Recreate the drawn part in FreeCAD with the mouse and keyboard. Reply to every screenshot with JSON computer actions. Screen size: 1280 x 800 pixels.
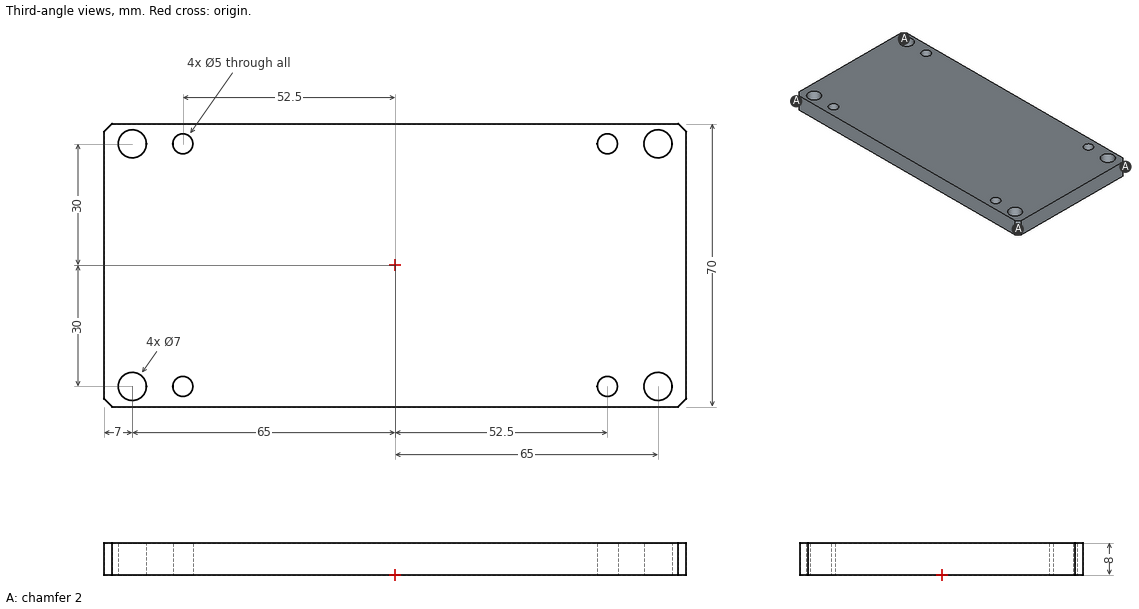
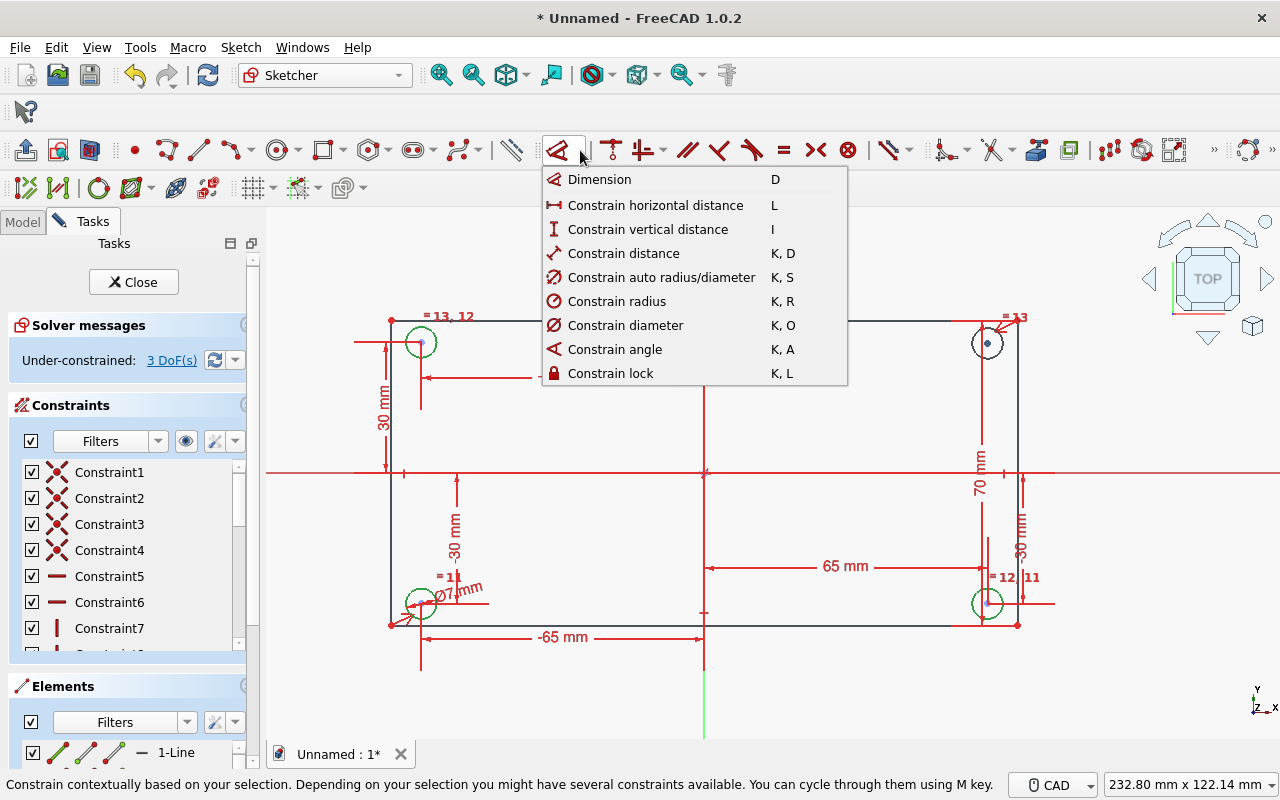
{"action": "left_click", "coordinate": [695, 205]}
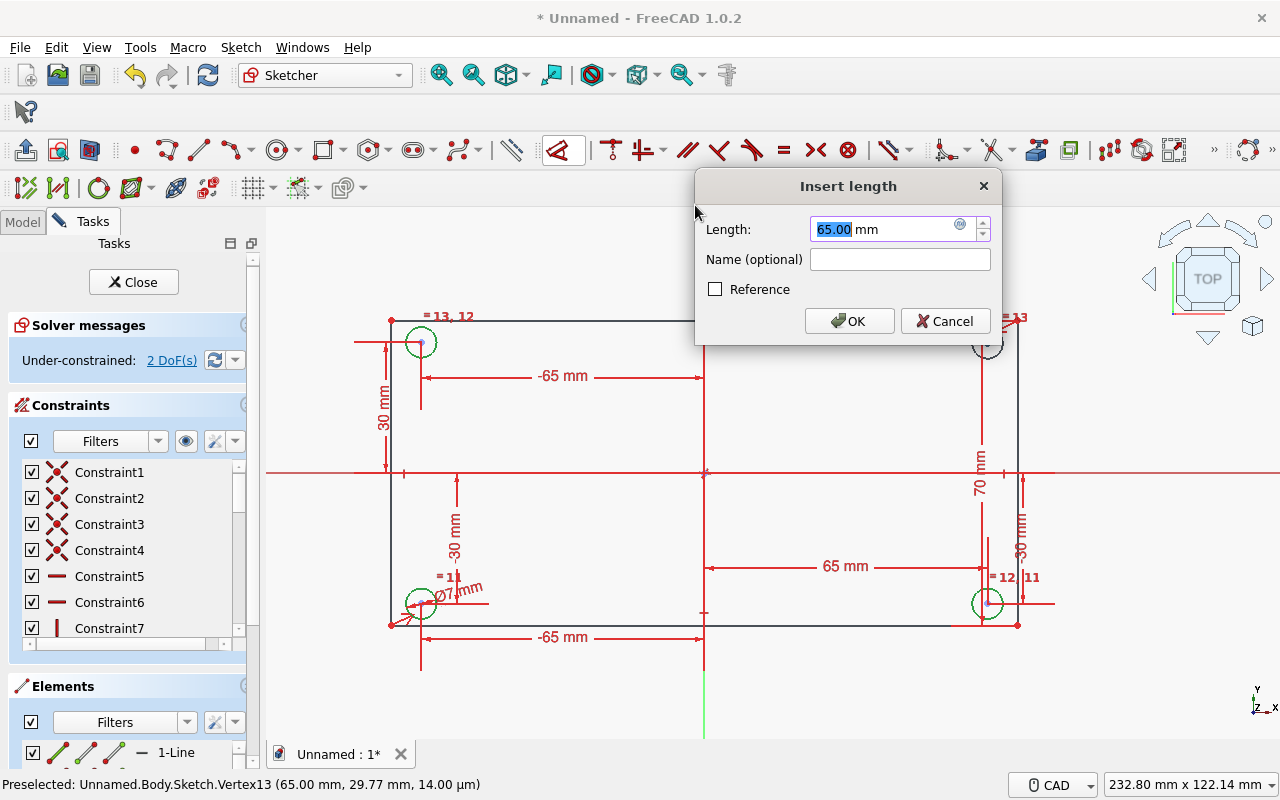
{"action": "type", "text": "65"}
{"action": "key", "text": "Return"}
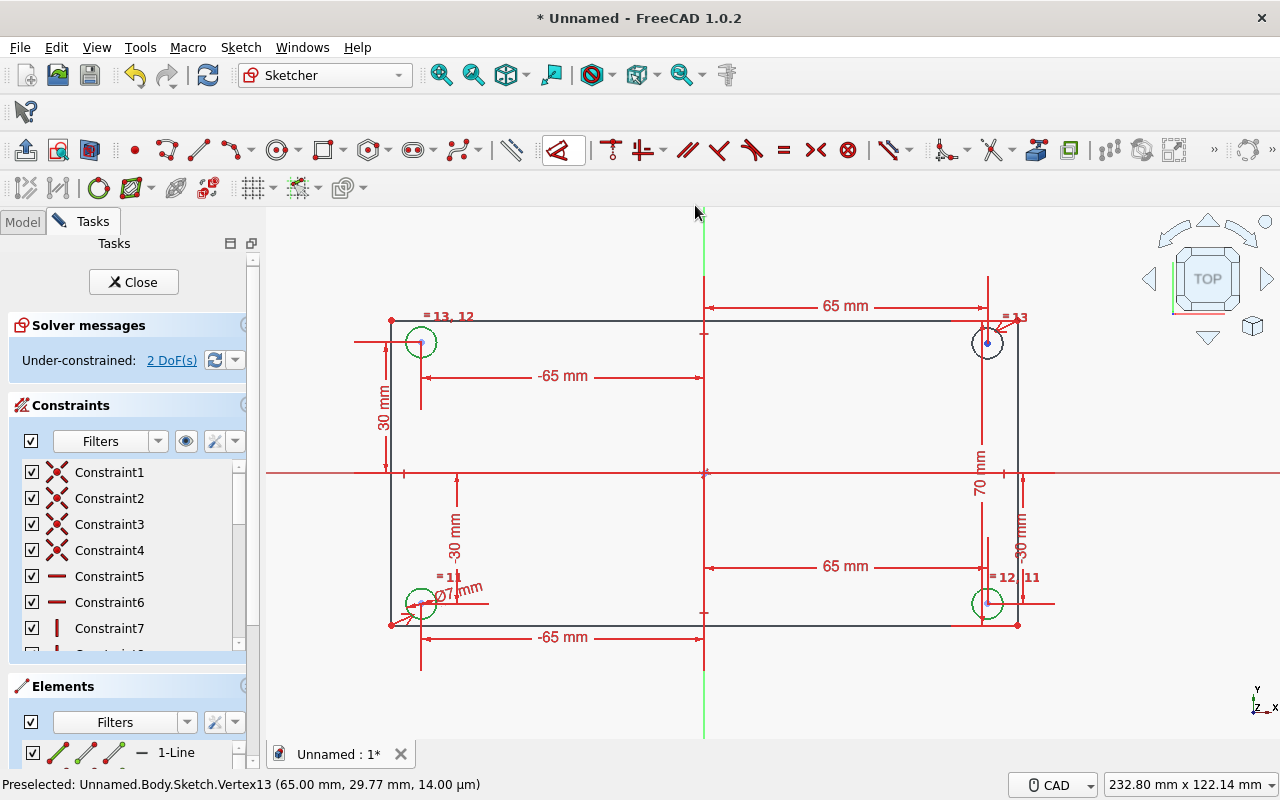
{"action": "left_click", "coordinate": [988, 343]}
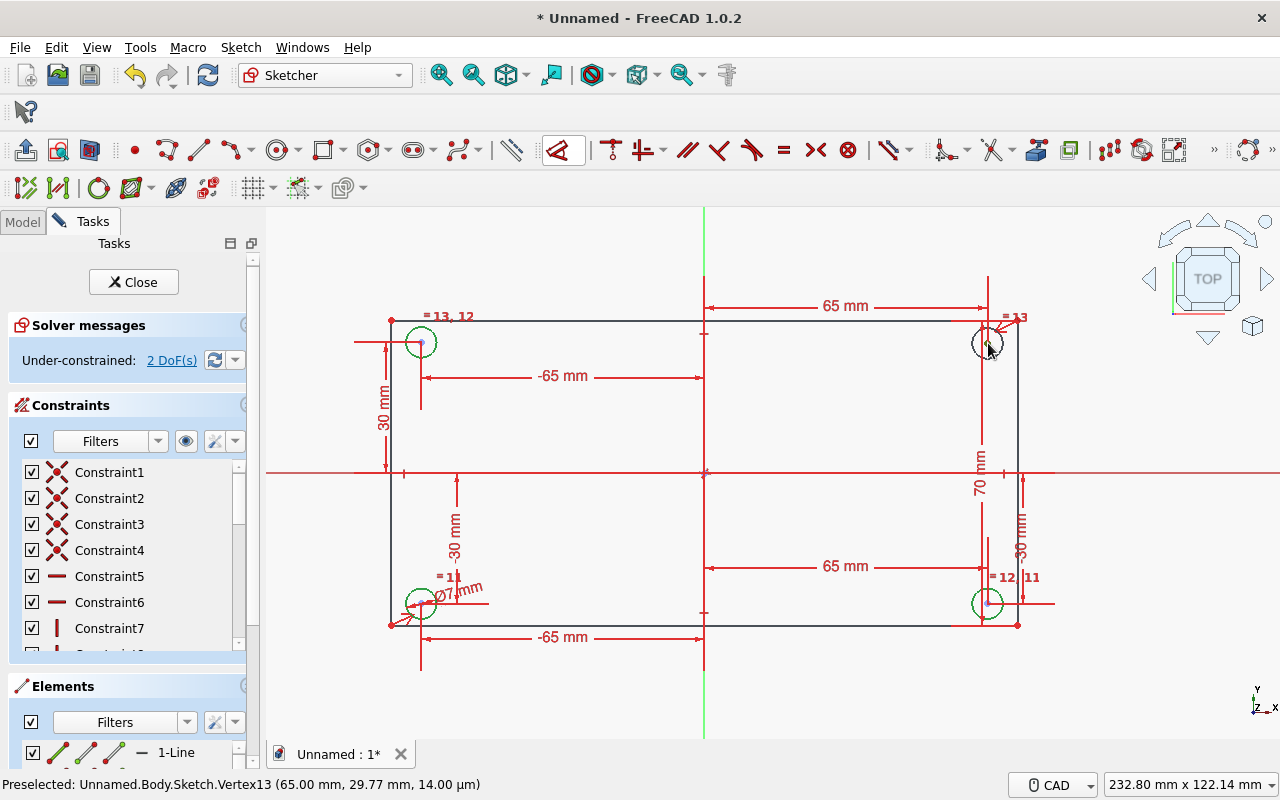
{"action": "key", "text": "i"}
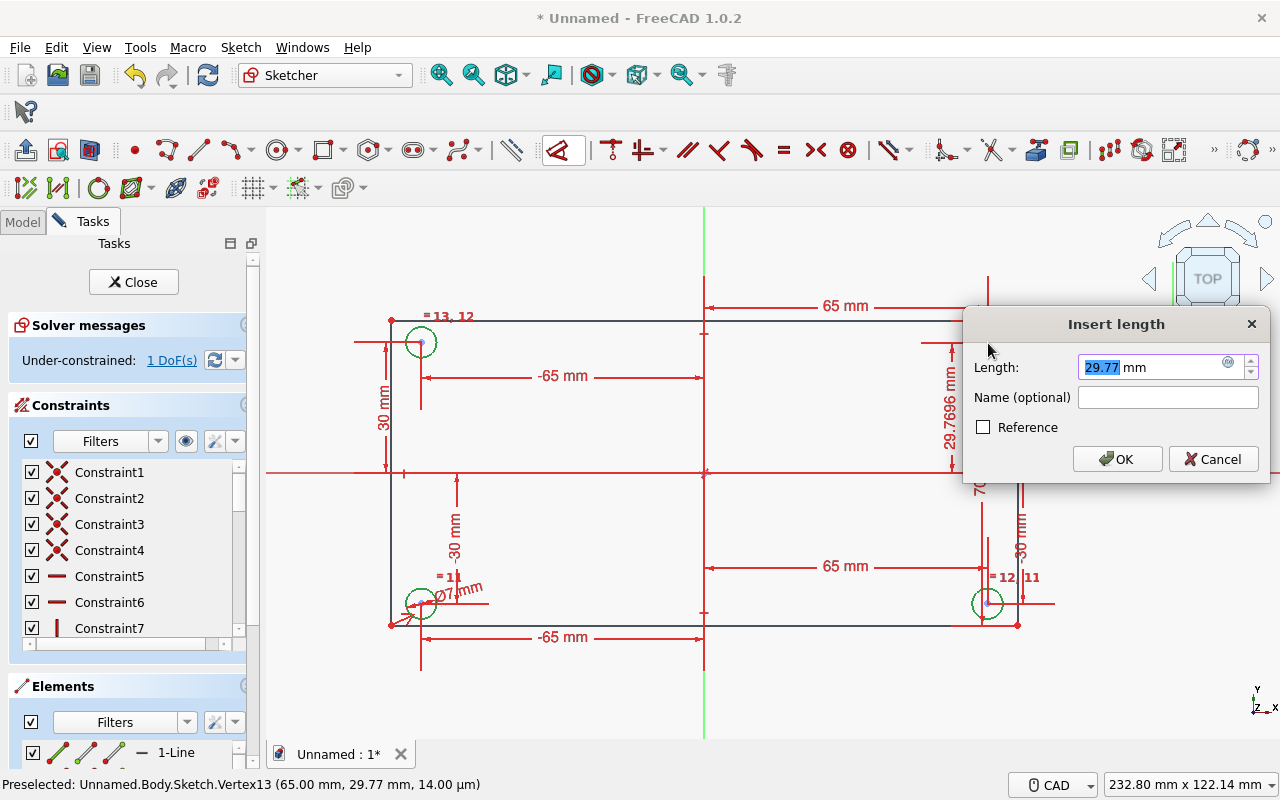
{"action": "type", "text": "30"}
{"action": "key", "text": "Return"}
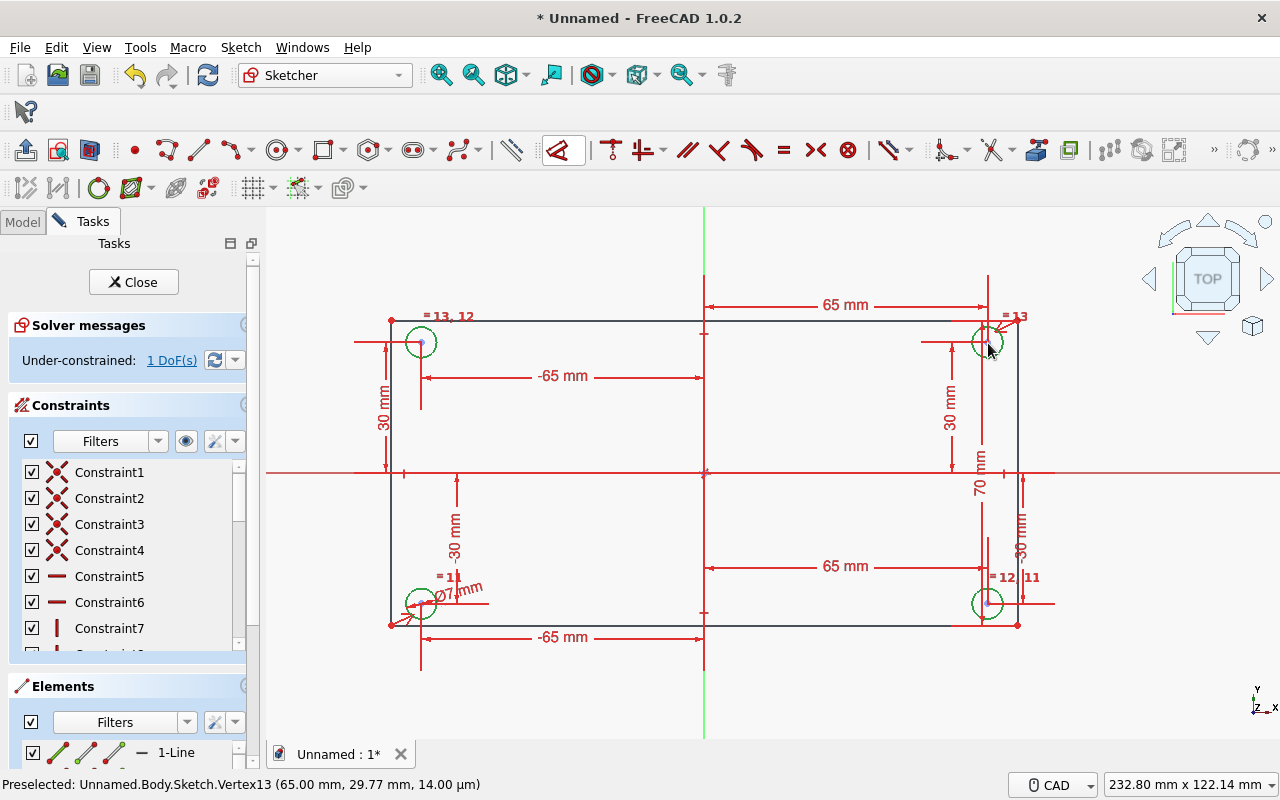
{"action": "scroll", "coordinate": [391, 626], "scroll_direction": "up", "scroll_amount": 2}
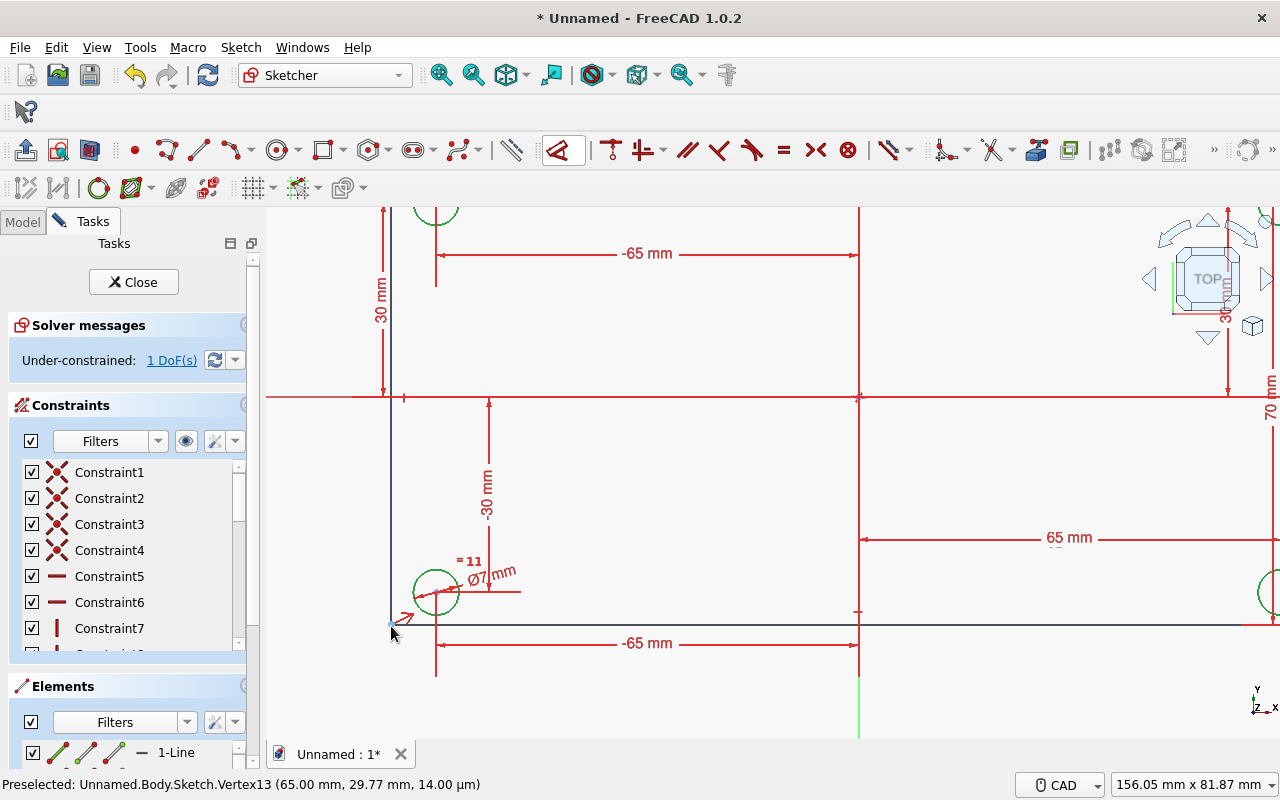
{"action": "left_click", "coordinate": [391, 625]}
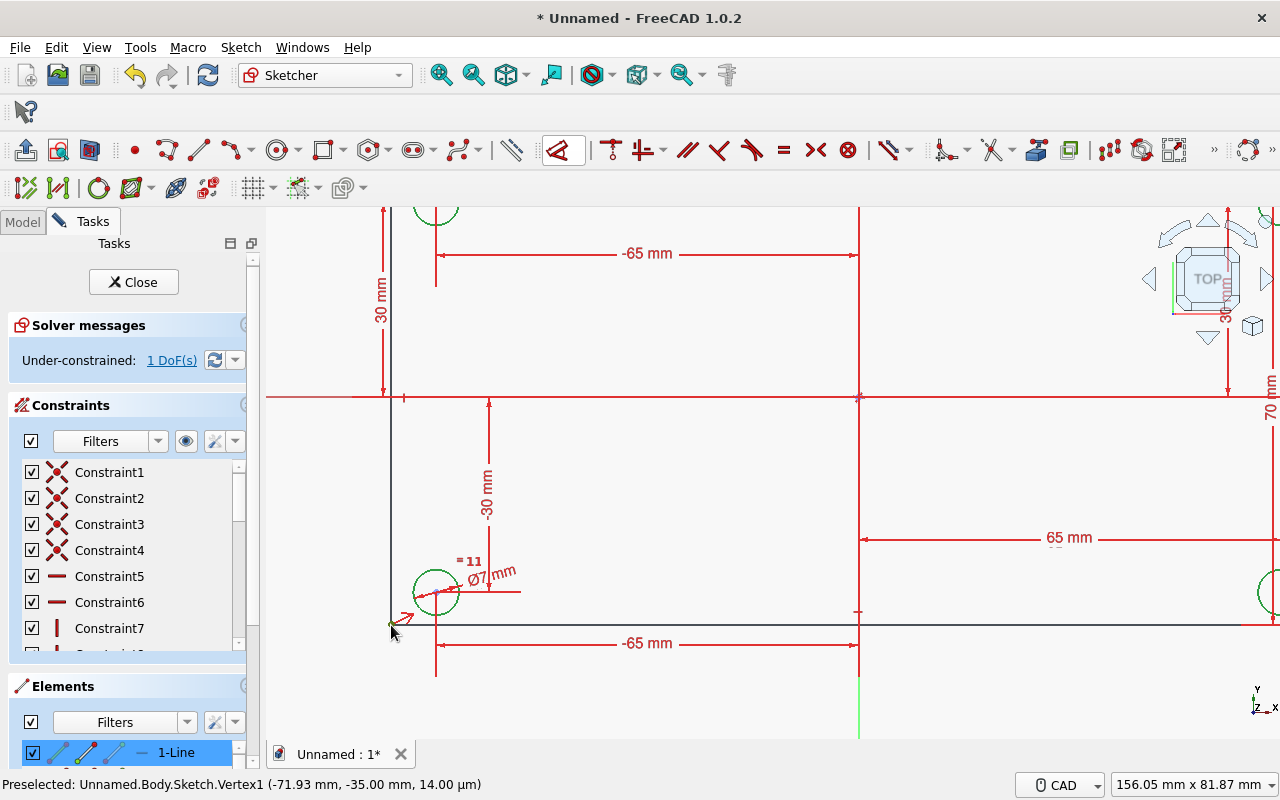
{"action": "left_click", "coordinate": [436, 592]}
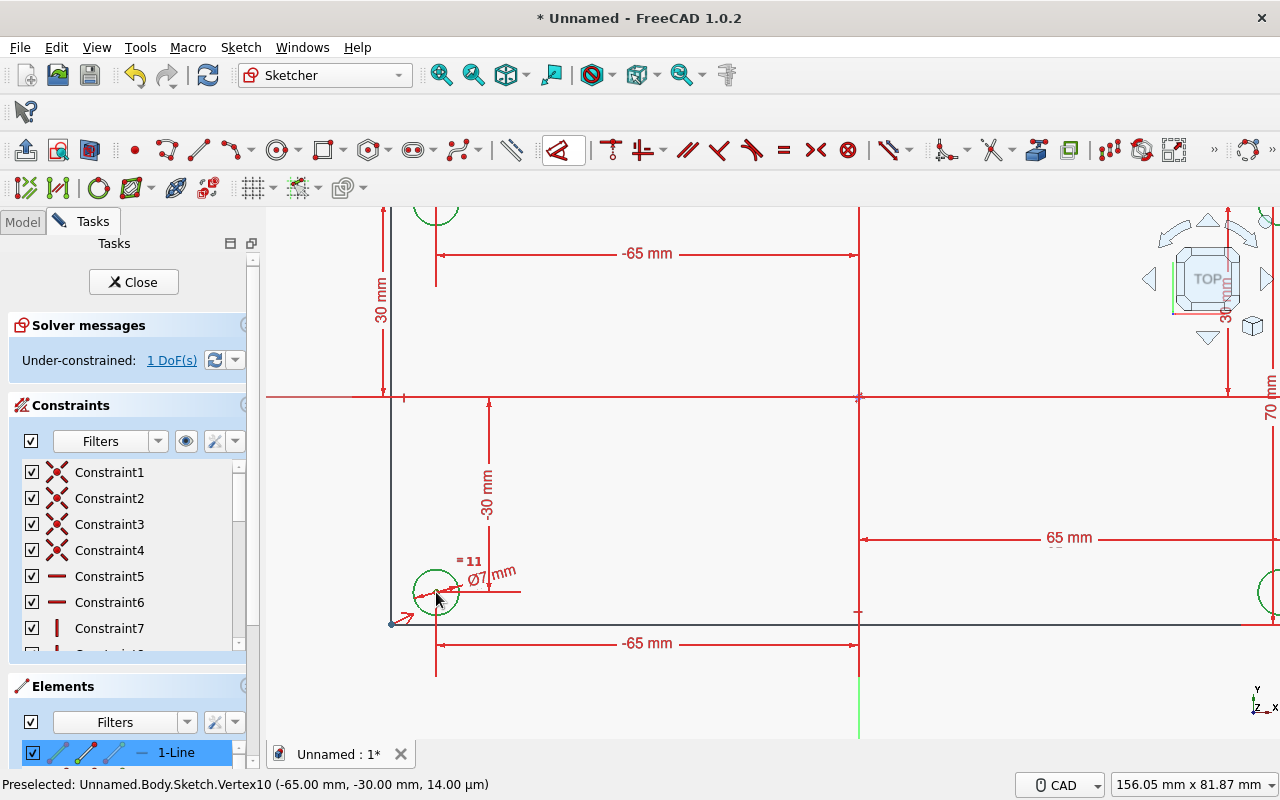
{"action": "key", "text": "l"}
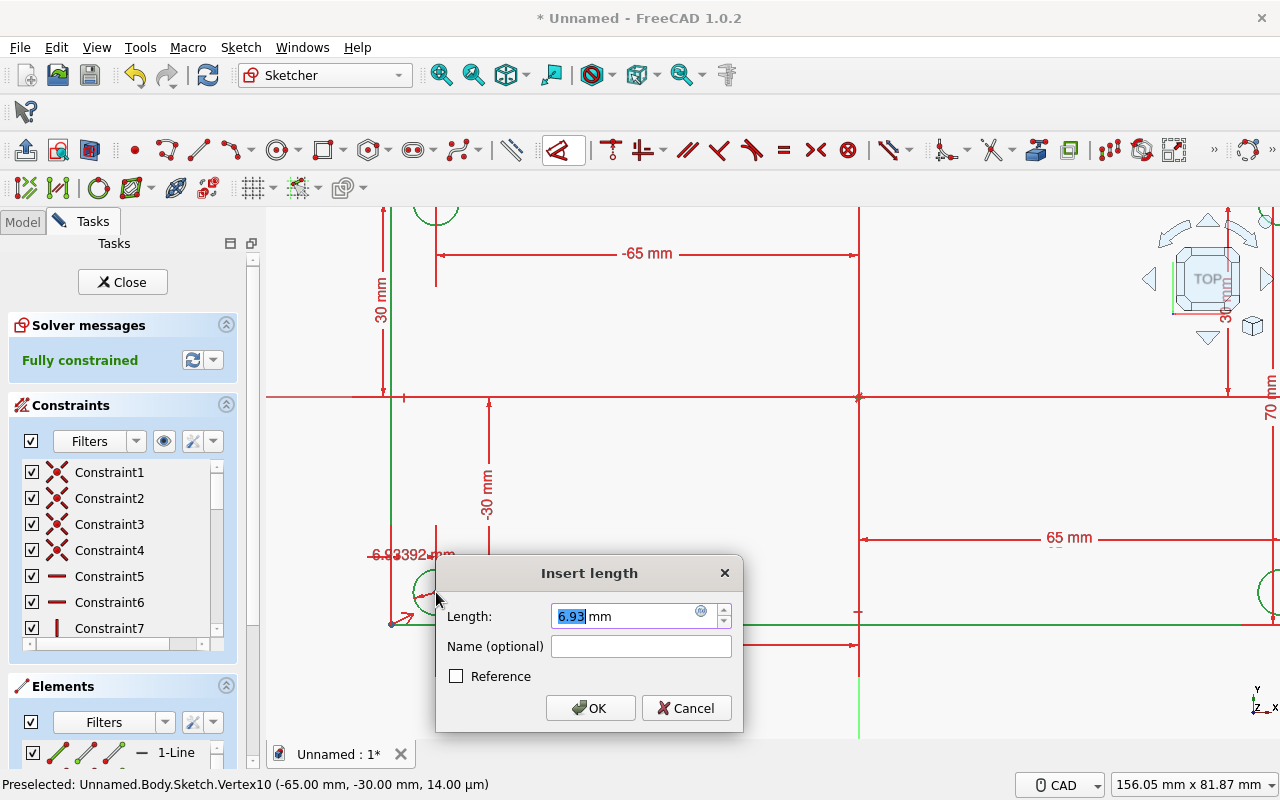
{"action": "type", "text": "7"}
{"action": "key", "text": "Return"}